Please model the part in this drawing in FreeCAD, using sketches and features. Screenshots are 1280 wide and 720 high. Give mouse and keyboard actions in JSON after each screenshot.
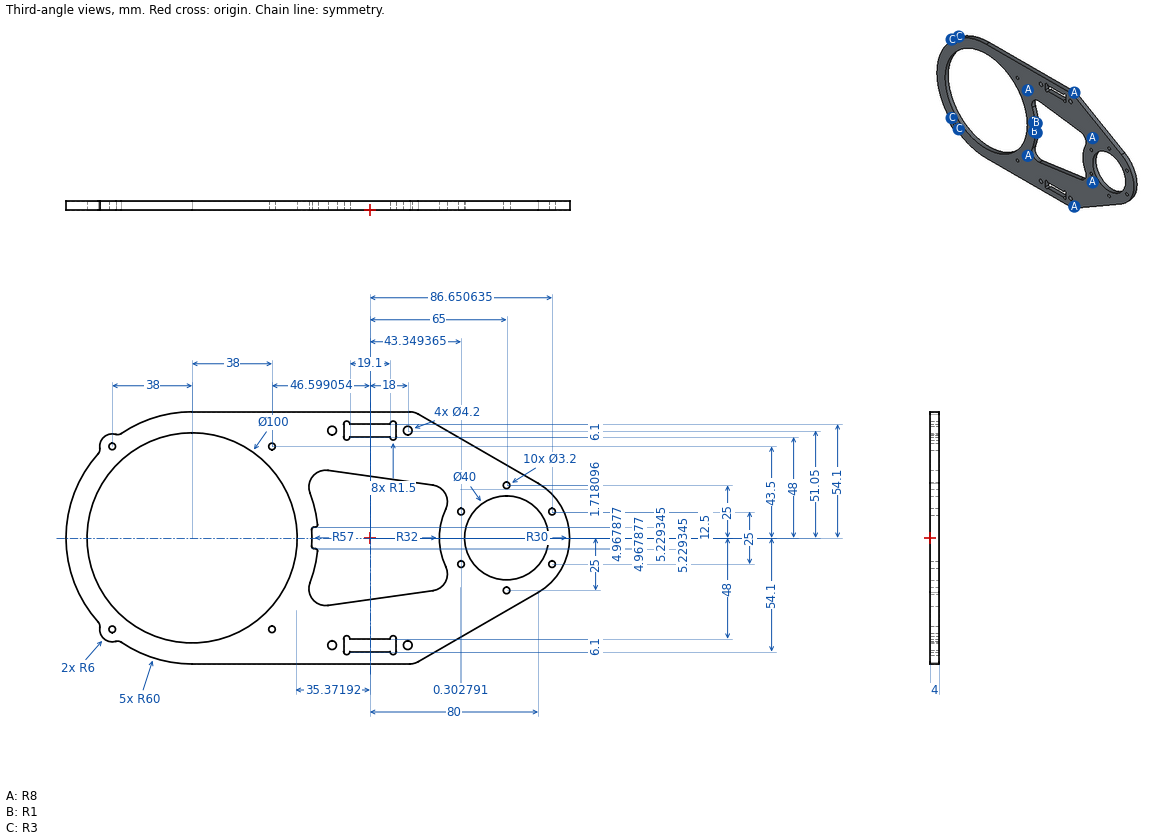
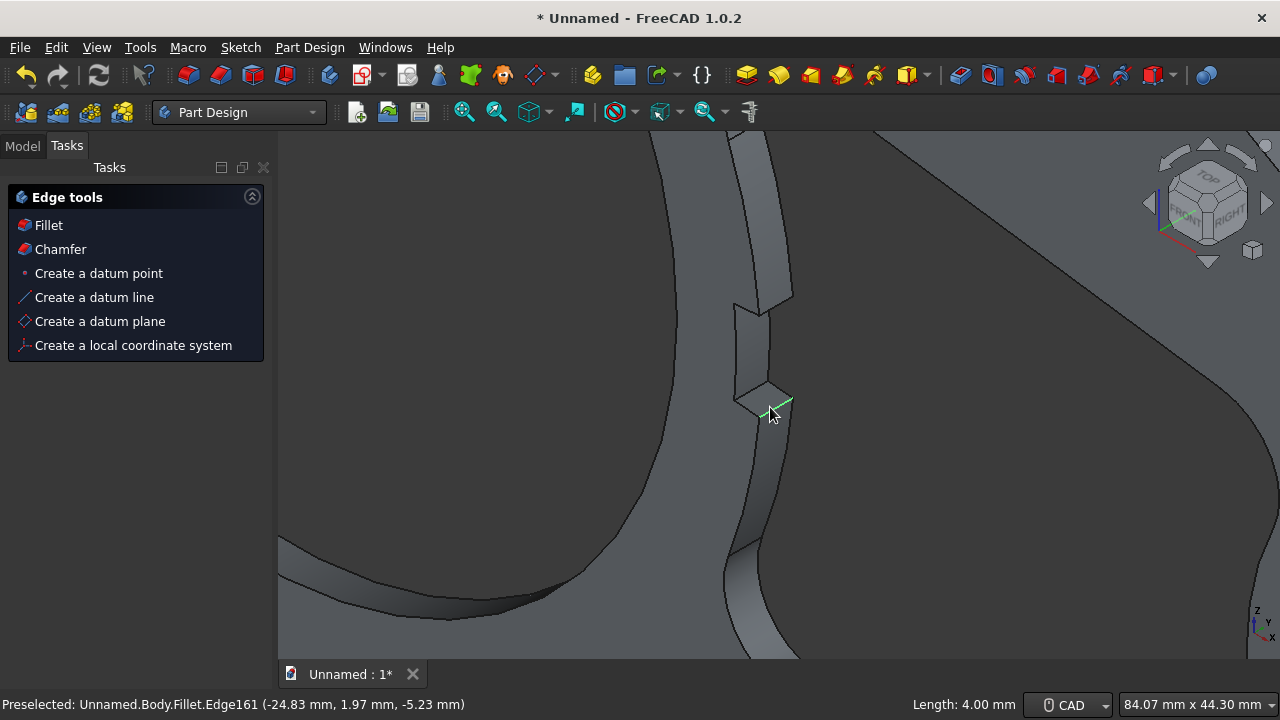
{"action": "key", "text": "v f"}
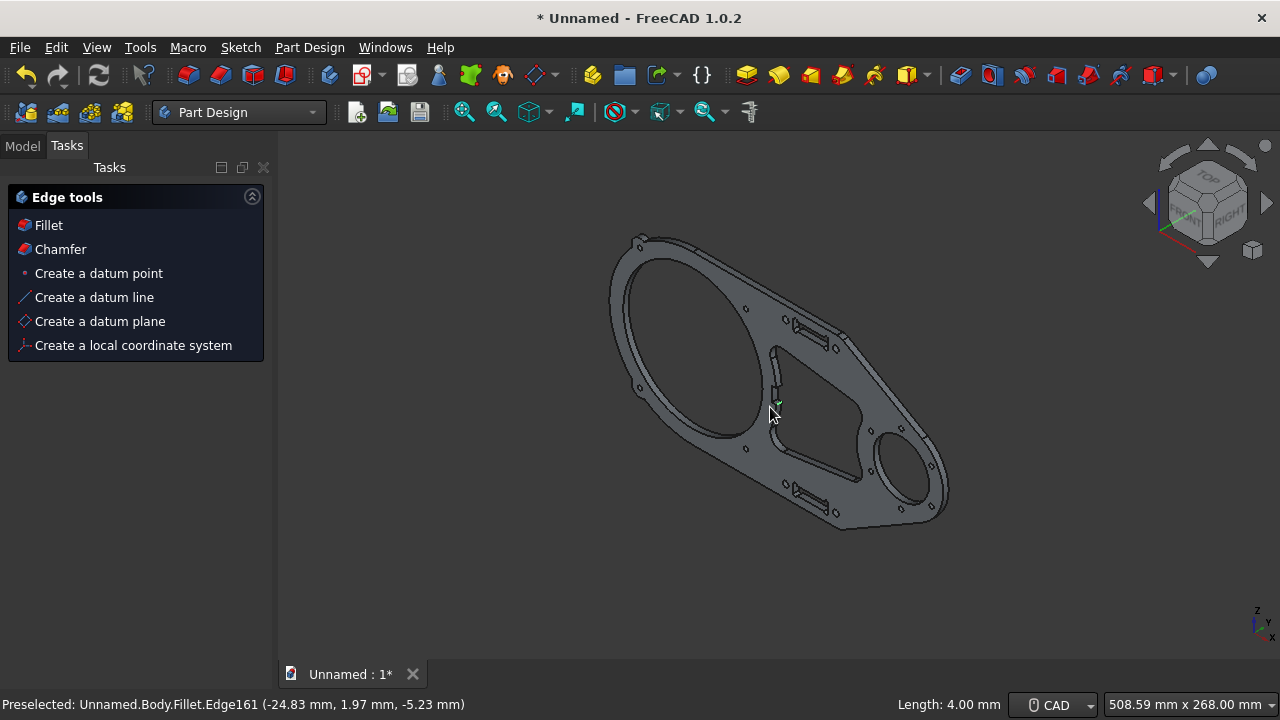
{"action": "key", "text": "2"}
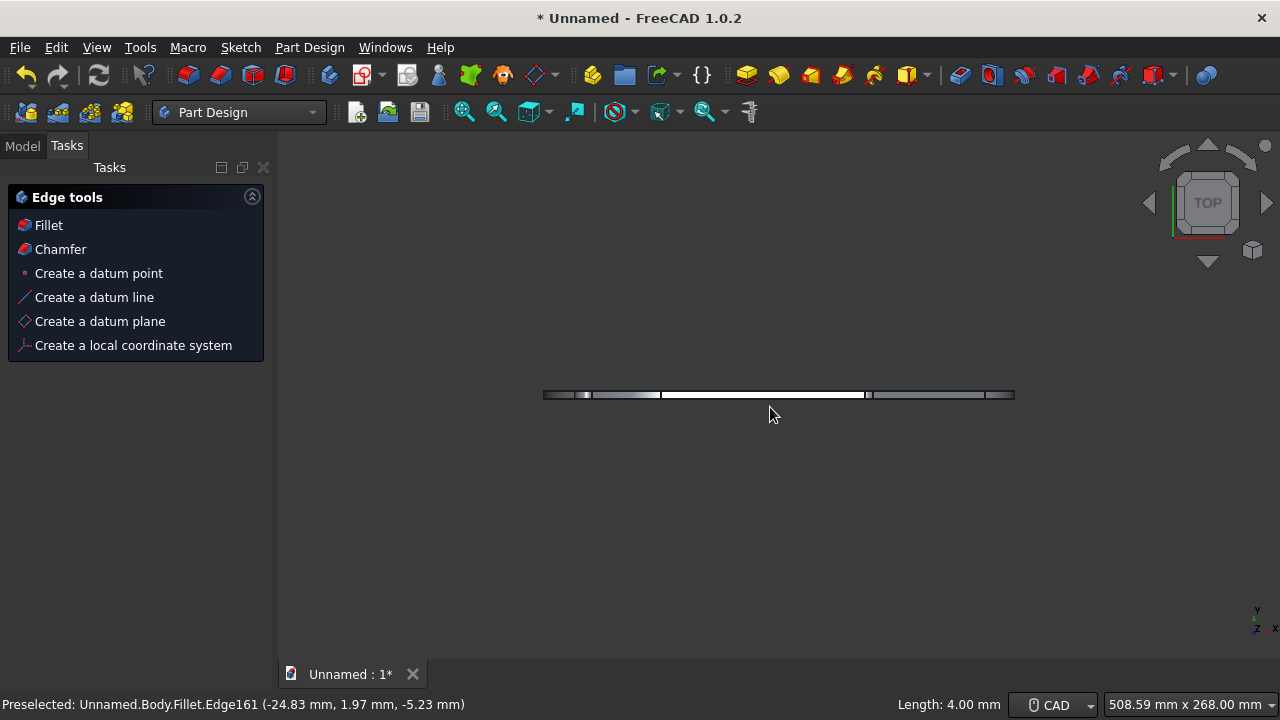
{"action": "scroll", "coordinate": [773, 394], "scroll_direction": "up", "scroll_amount": 9}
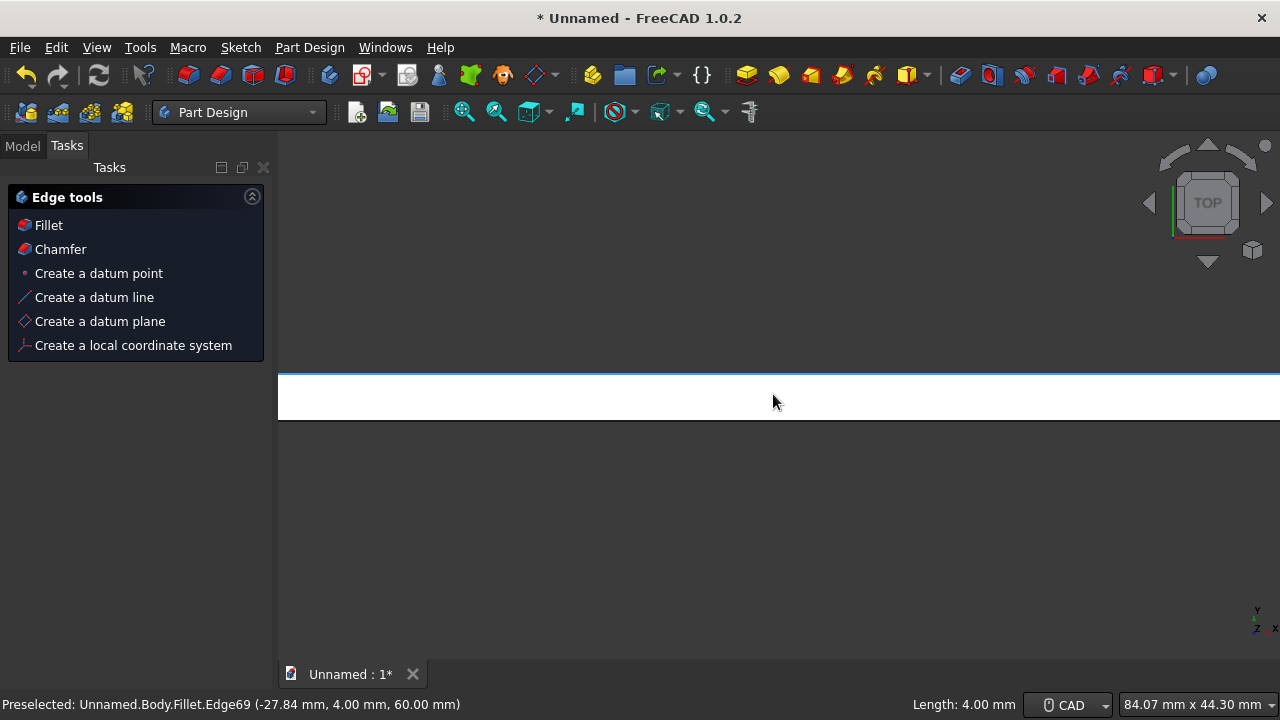
{"action": "left_click", "coordinate": [466, 112]}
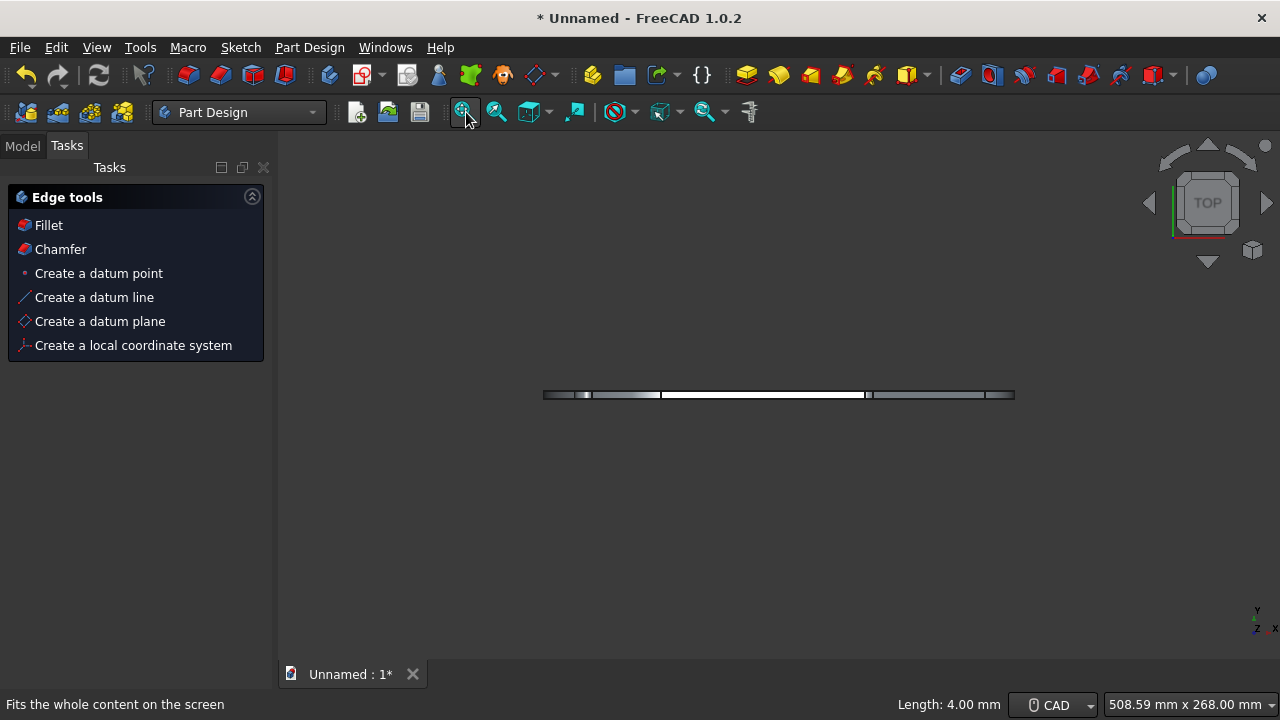
{"action": "key", "text": "1"}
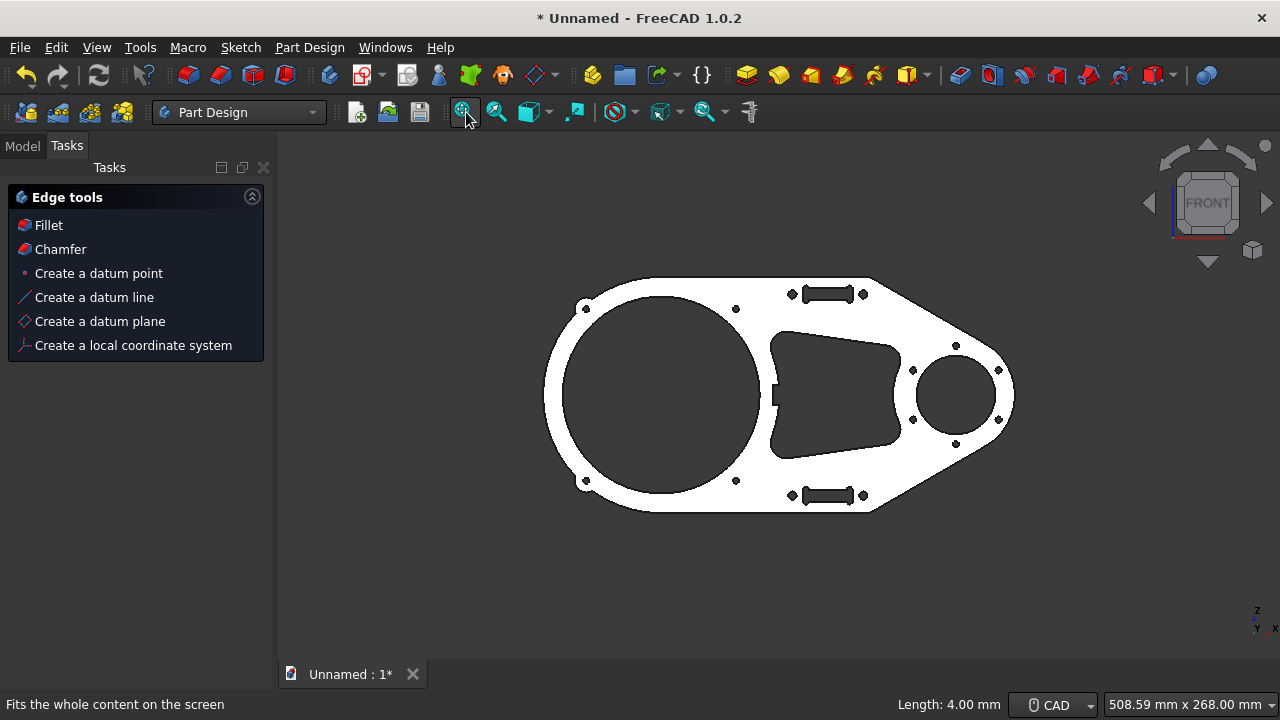
{"action": "scroll", "coordinate": [773, 404], "scroll_direction": "up", "scroll_amount": 9}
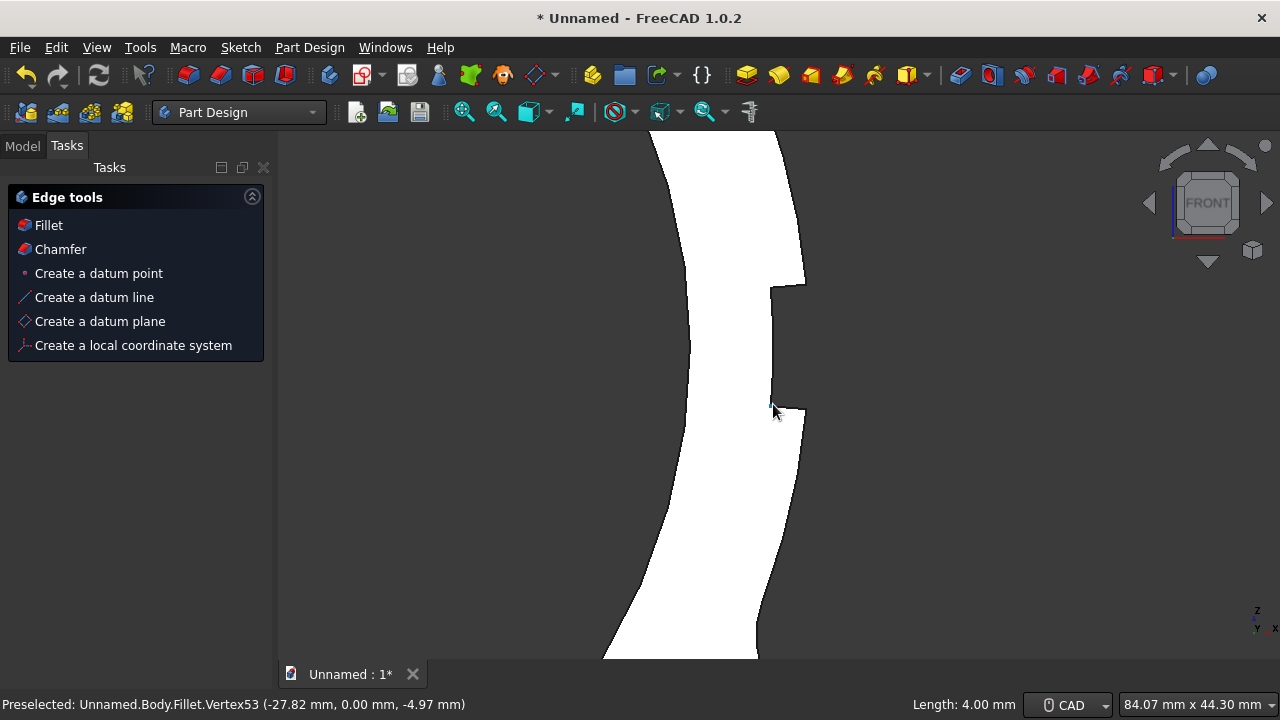
{"action": "left_click", "coordinate": [466, 112]}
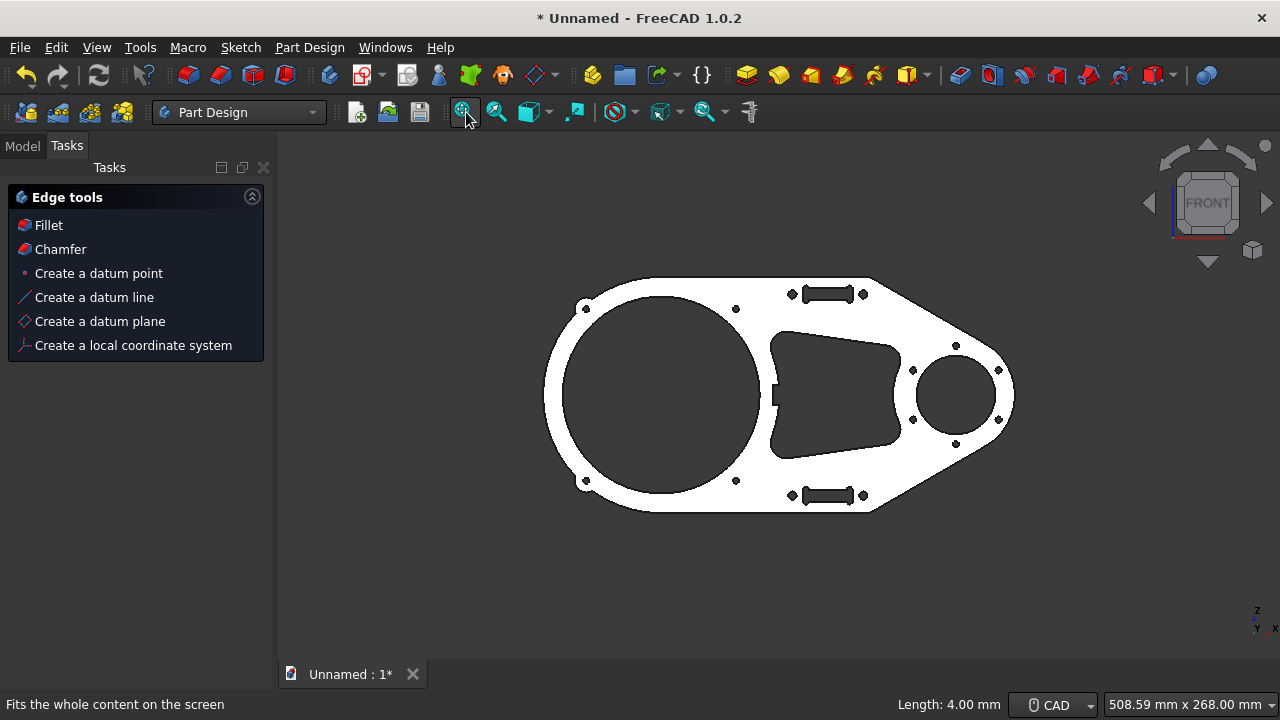
{"action": "key", "text": "3"}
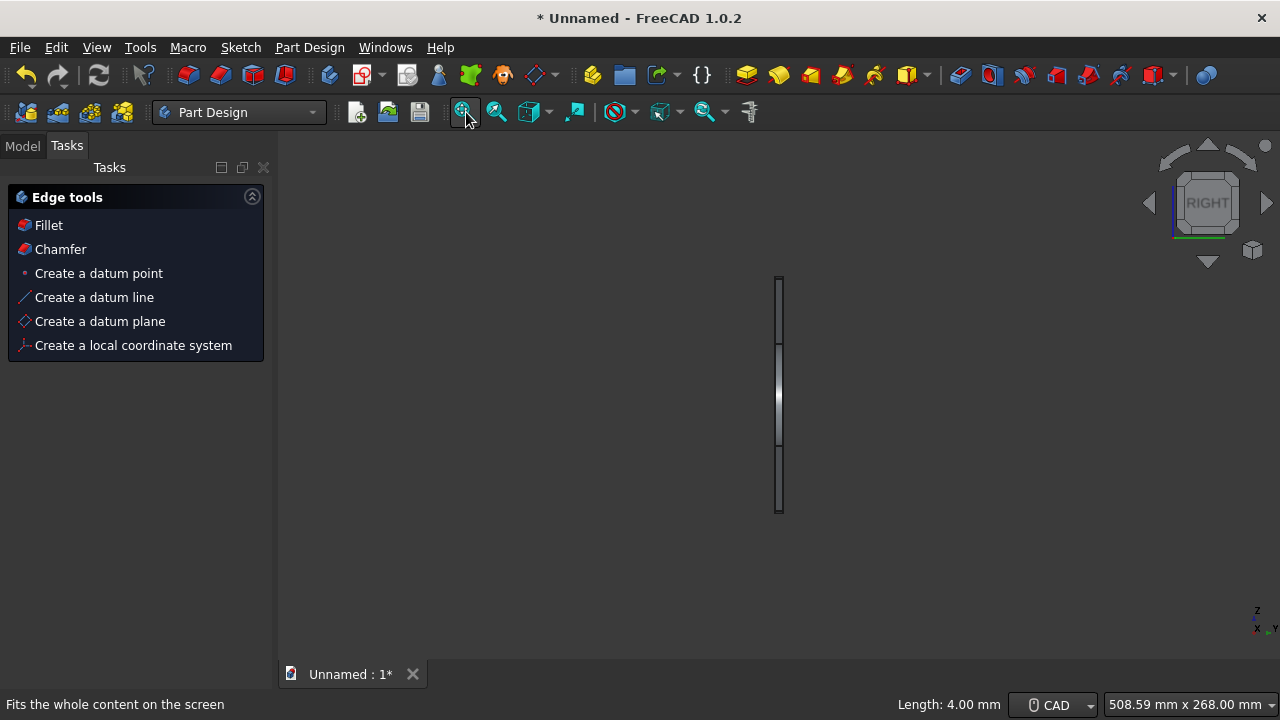
{"action": "left_click", "coordinate": [466, 112]}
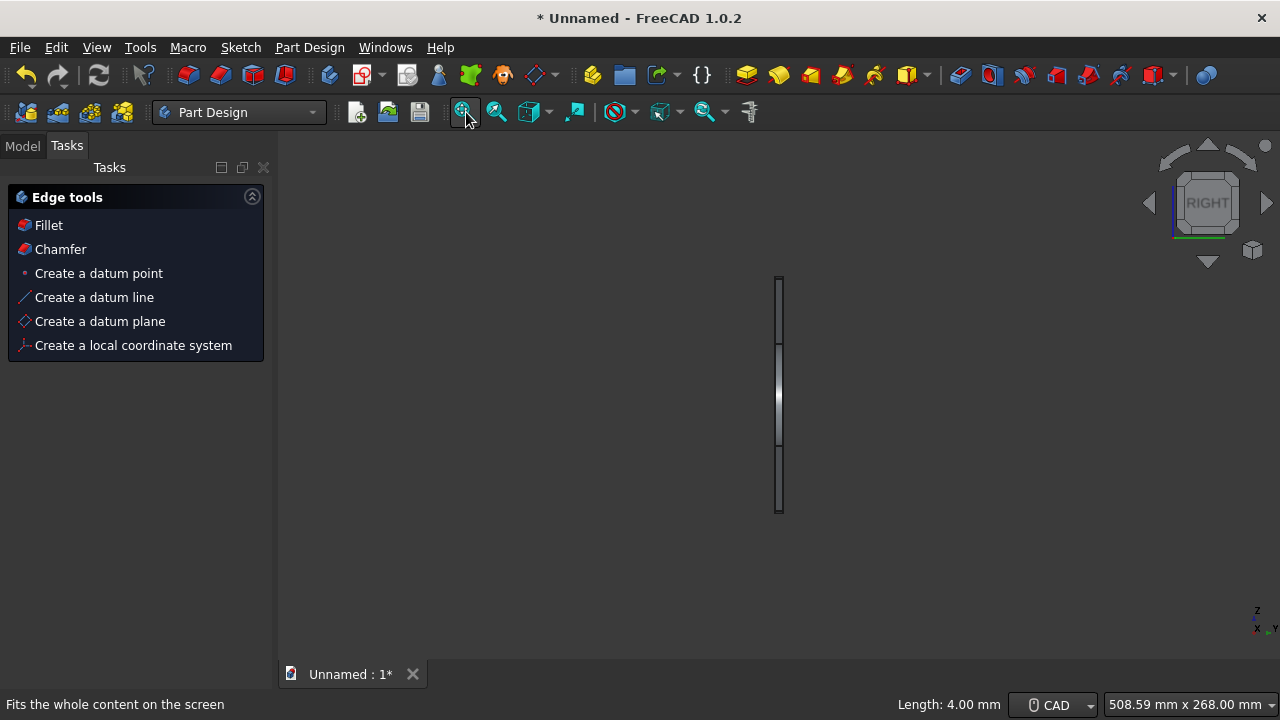
{"action": "scroll", "coordinate": [779, 404], "scroll_direction": "up", "scroll_amount": 9}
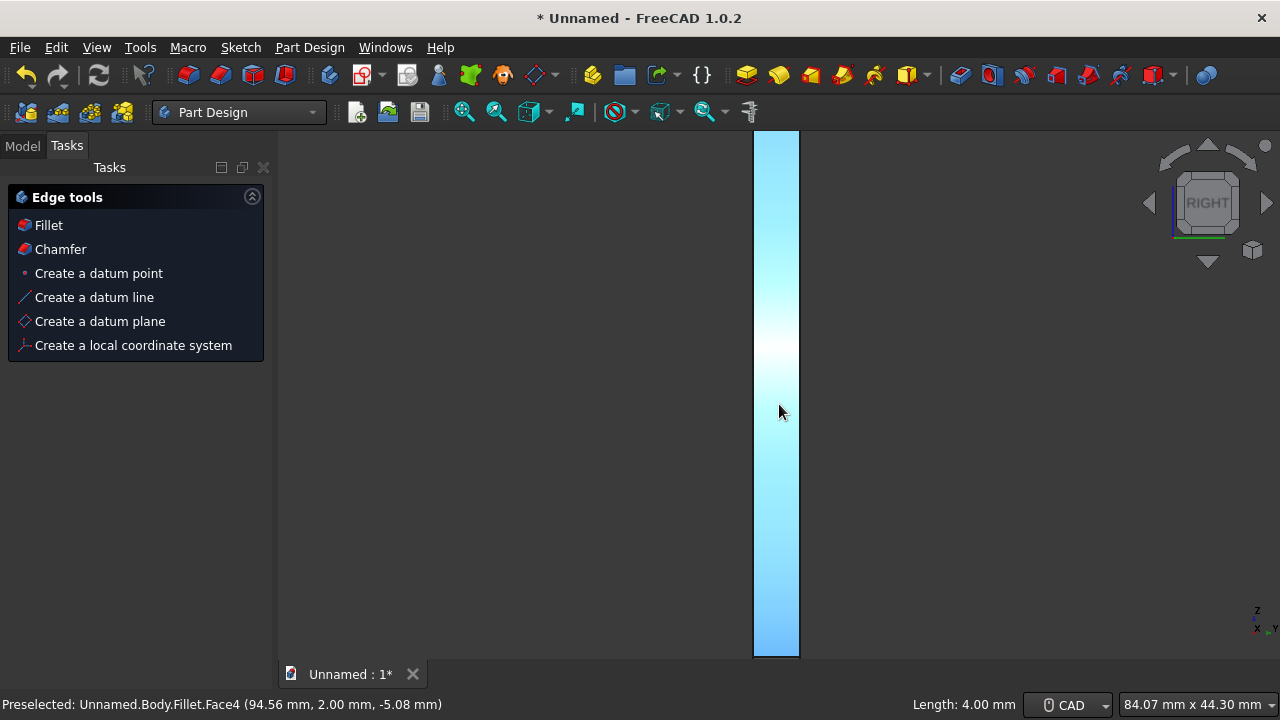
{"action": "left_click", "coordinate": [466, 112]}